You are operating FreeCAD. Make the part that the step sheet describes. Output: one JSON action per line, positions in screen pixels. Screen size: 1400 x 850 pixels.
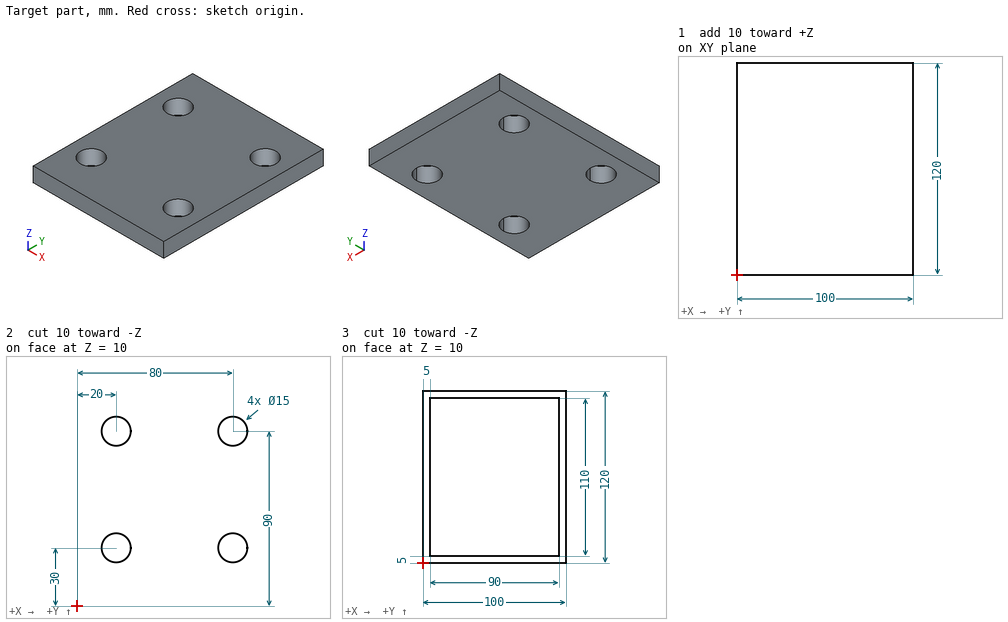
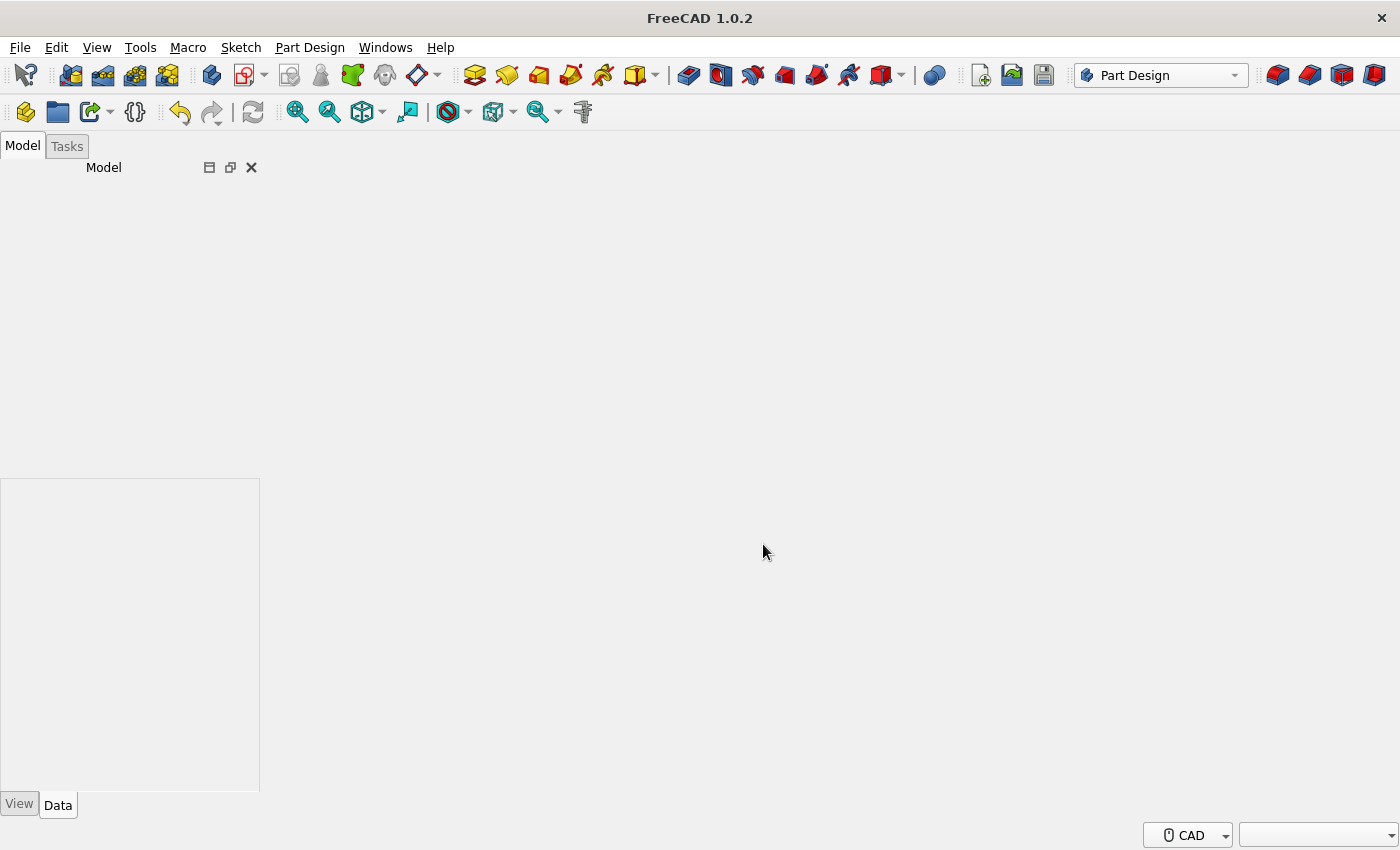
{"action": "key", "text": "ctrl+n"}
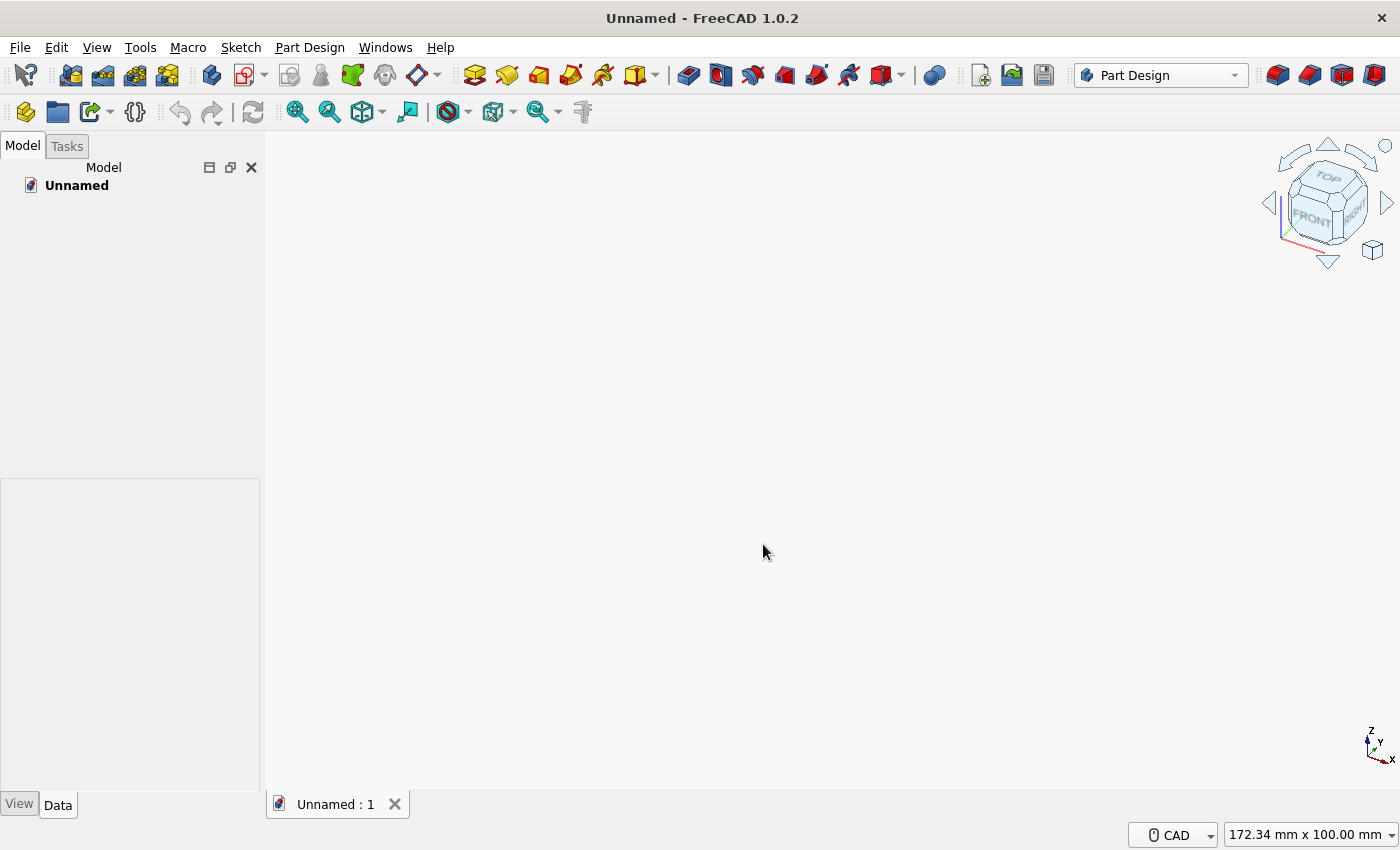
{"action": "left_click", "coordinate": [244, 76]}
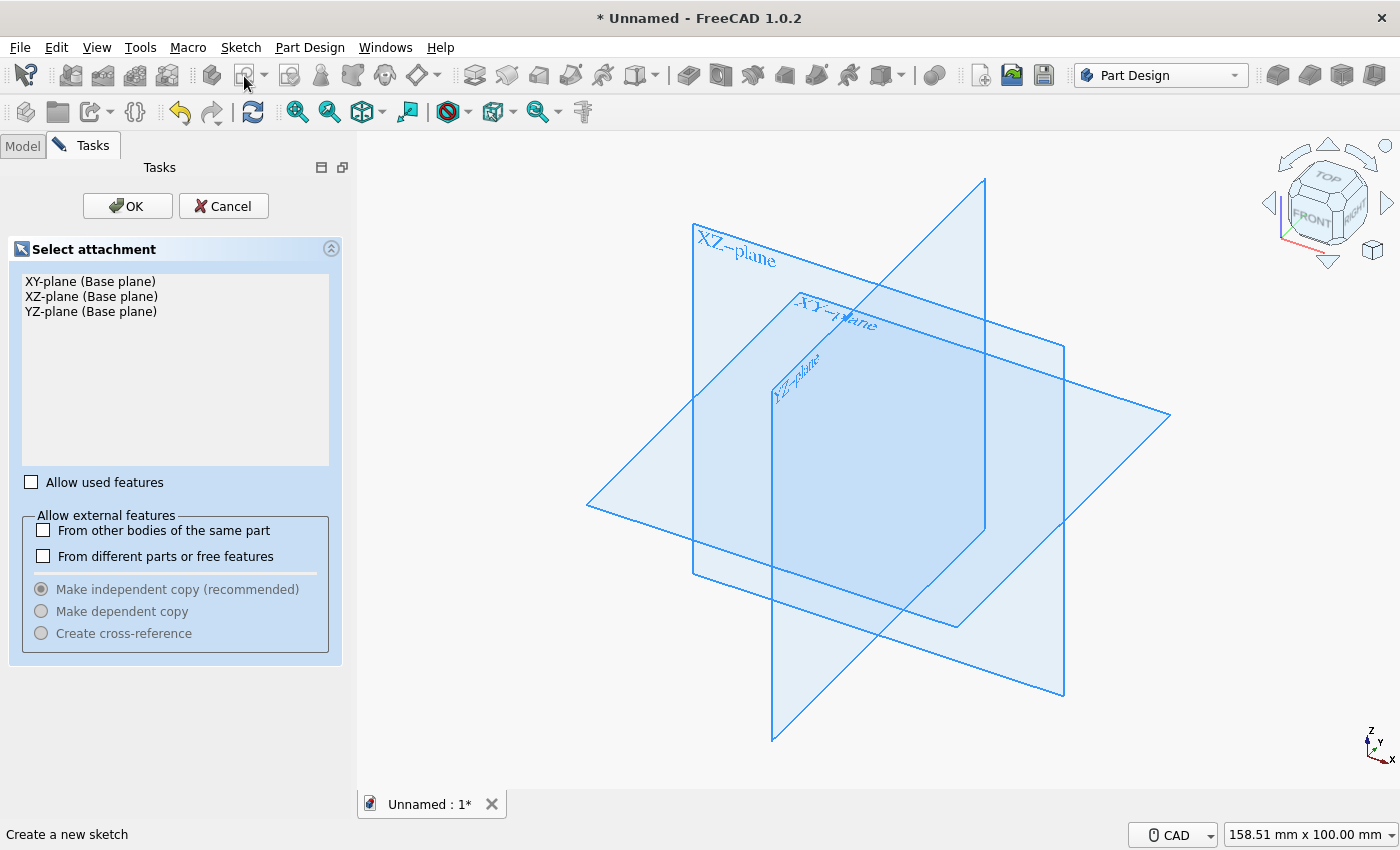
{"action": "left_click", "coordinate": [82, 282]}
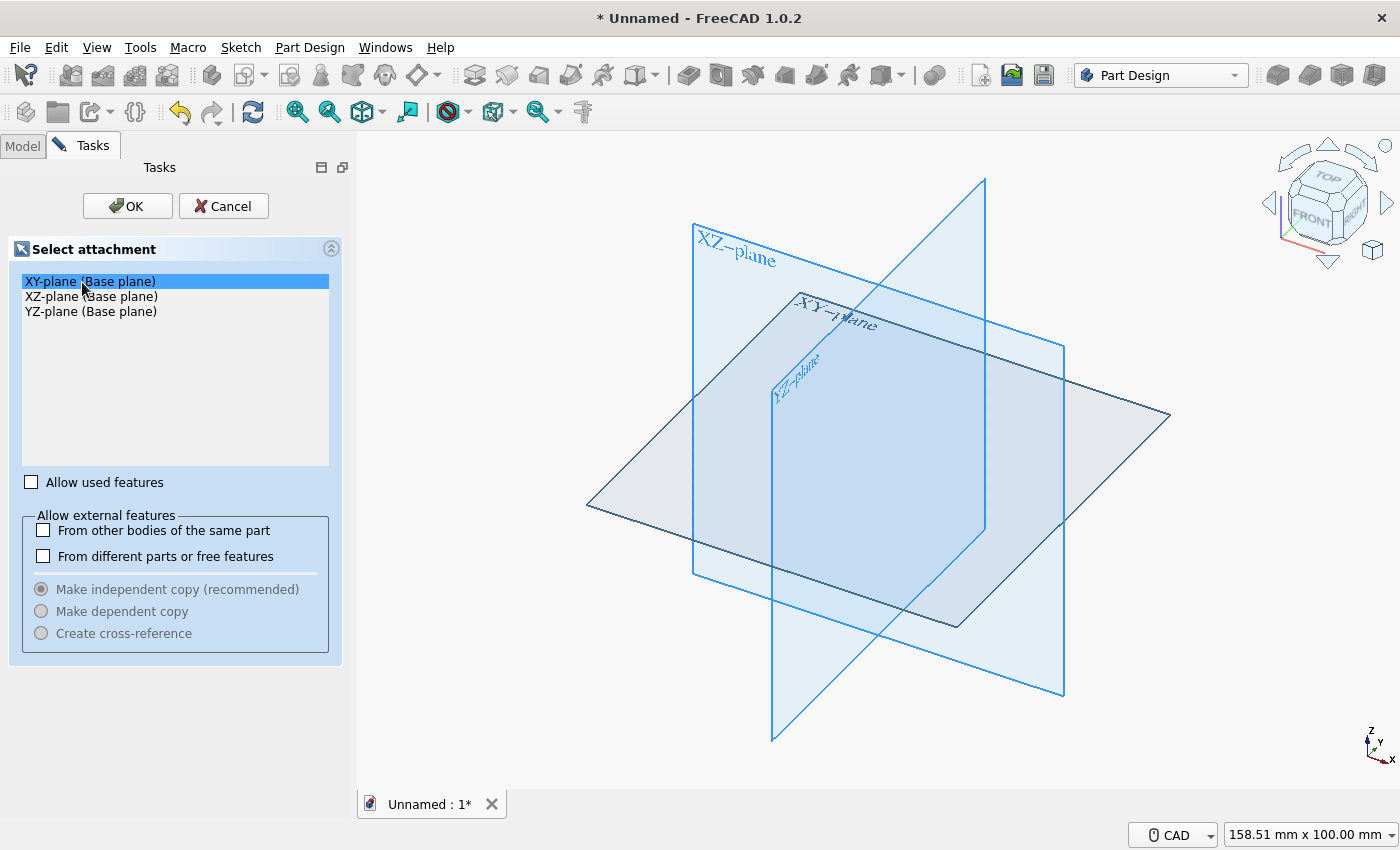
{"action": "left_click", "coordinate": [128, 206]}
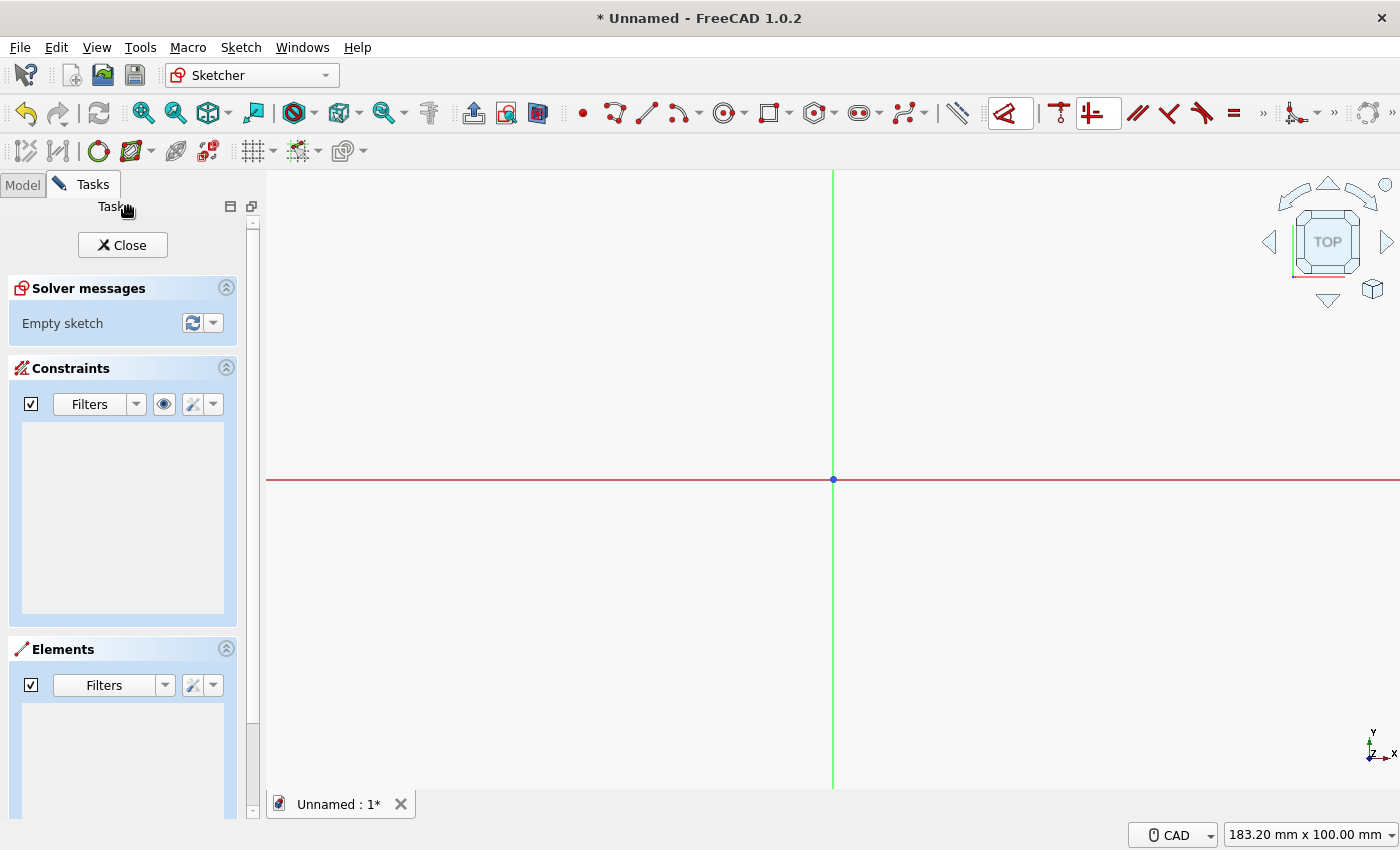
{"action": "scroll", "coordinate": [456, 761], "scroll_direction": "down", "scroll_amount": 4}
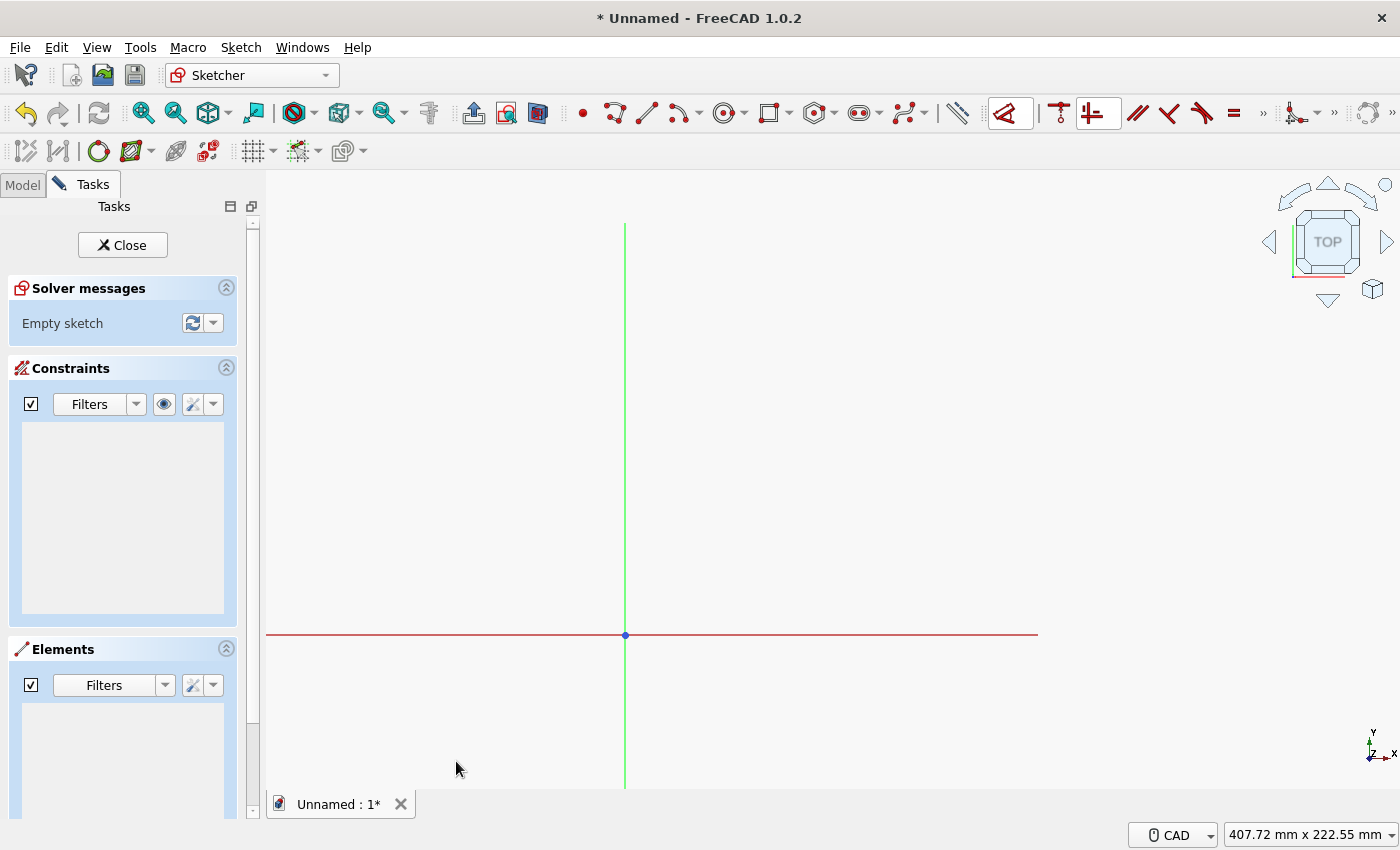
{"action": "key", "text": "g r"}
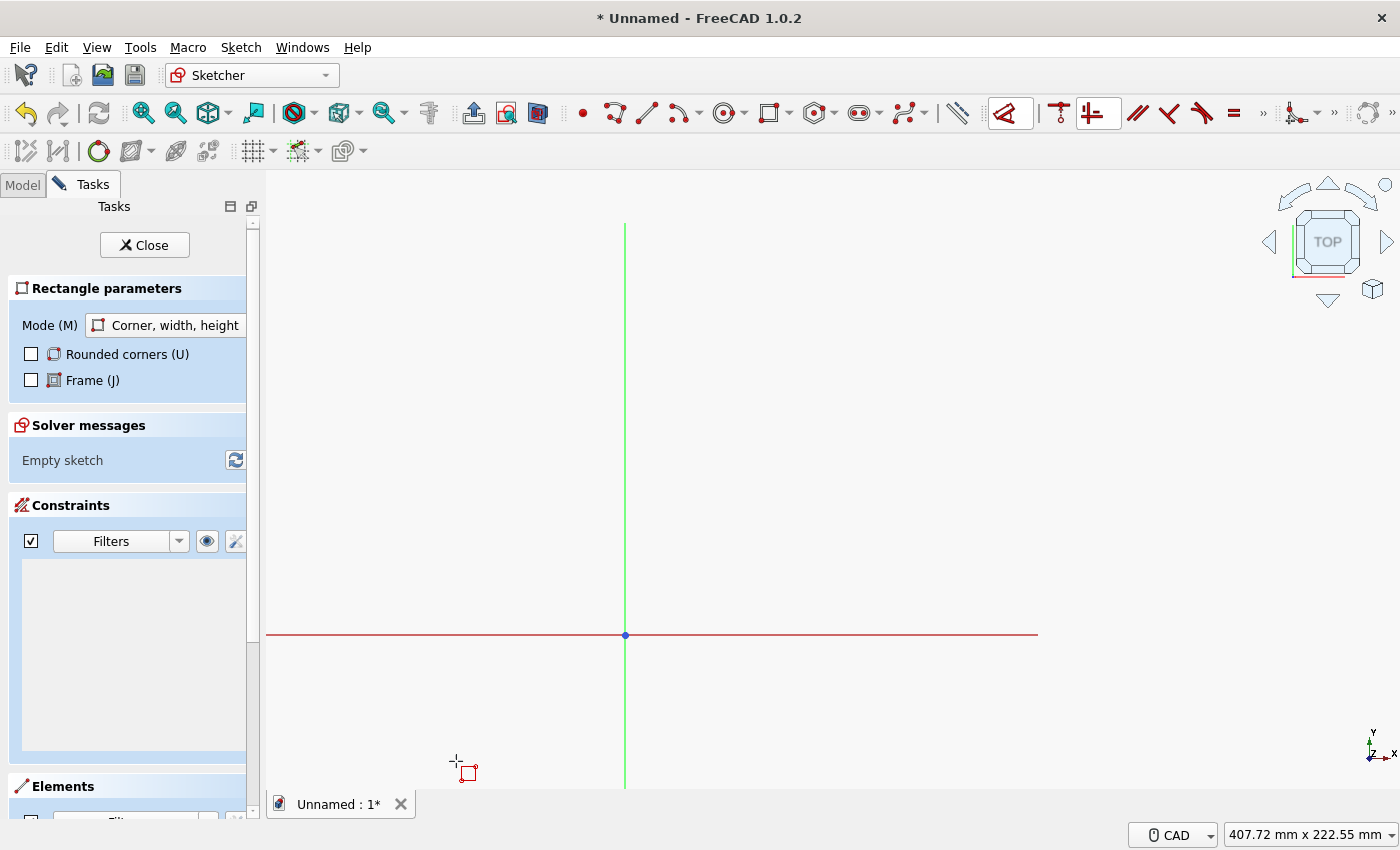
{"action": "left_click", "coordinate": [625, 635]}
{"action": "mouse_move", "coordinate": [904, 301]}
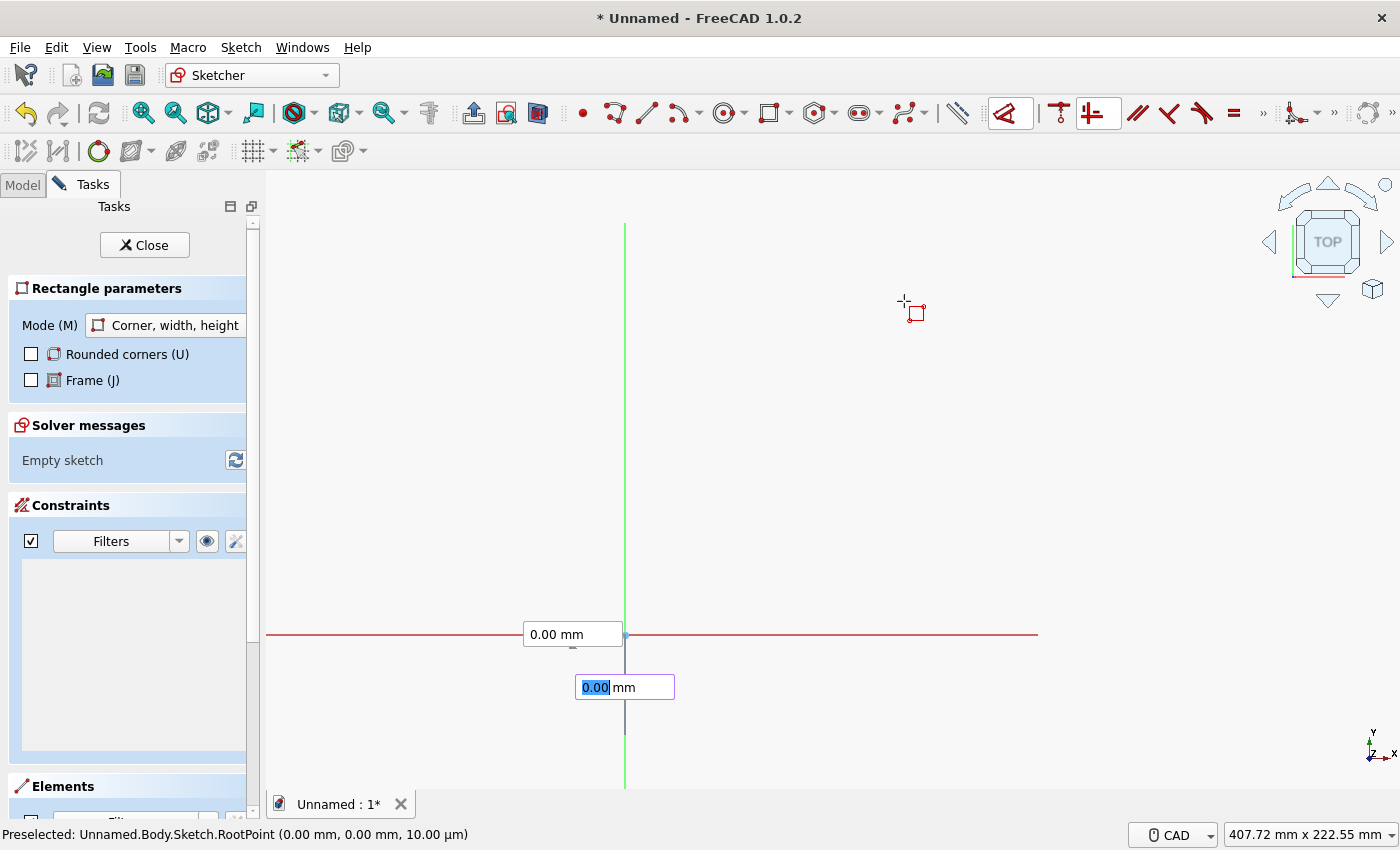
{"action": "type", "text": "100"}
{"action": "key", "text": "Tab"}
{"action": "type", "text": "120"}
{"action": "key", "text": "Return"}
{"action": "key", "text": "Escape"}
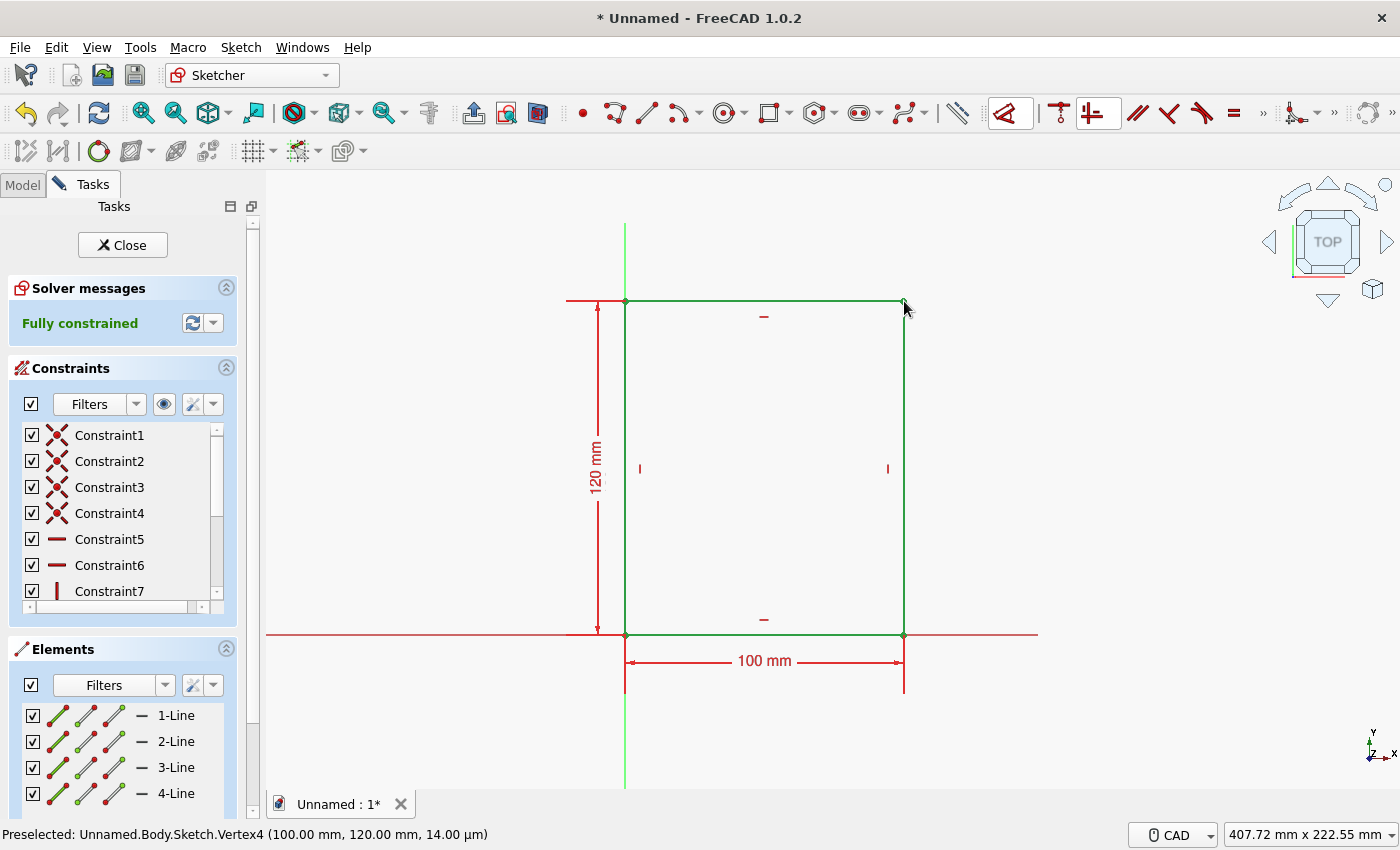
{"action": "left_click", "coordinate": [123, 245]}